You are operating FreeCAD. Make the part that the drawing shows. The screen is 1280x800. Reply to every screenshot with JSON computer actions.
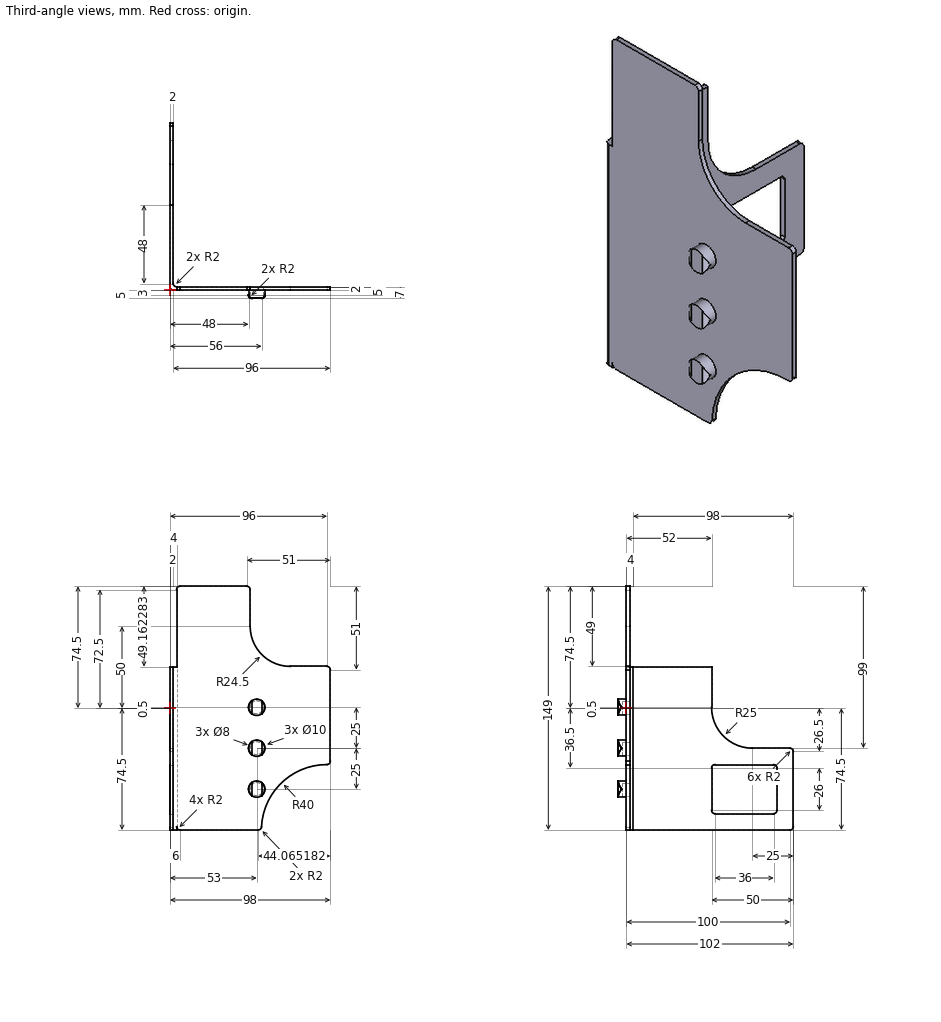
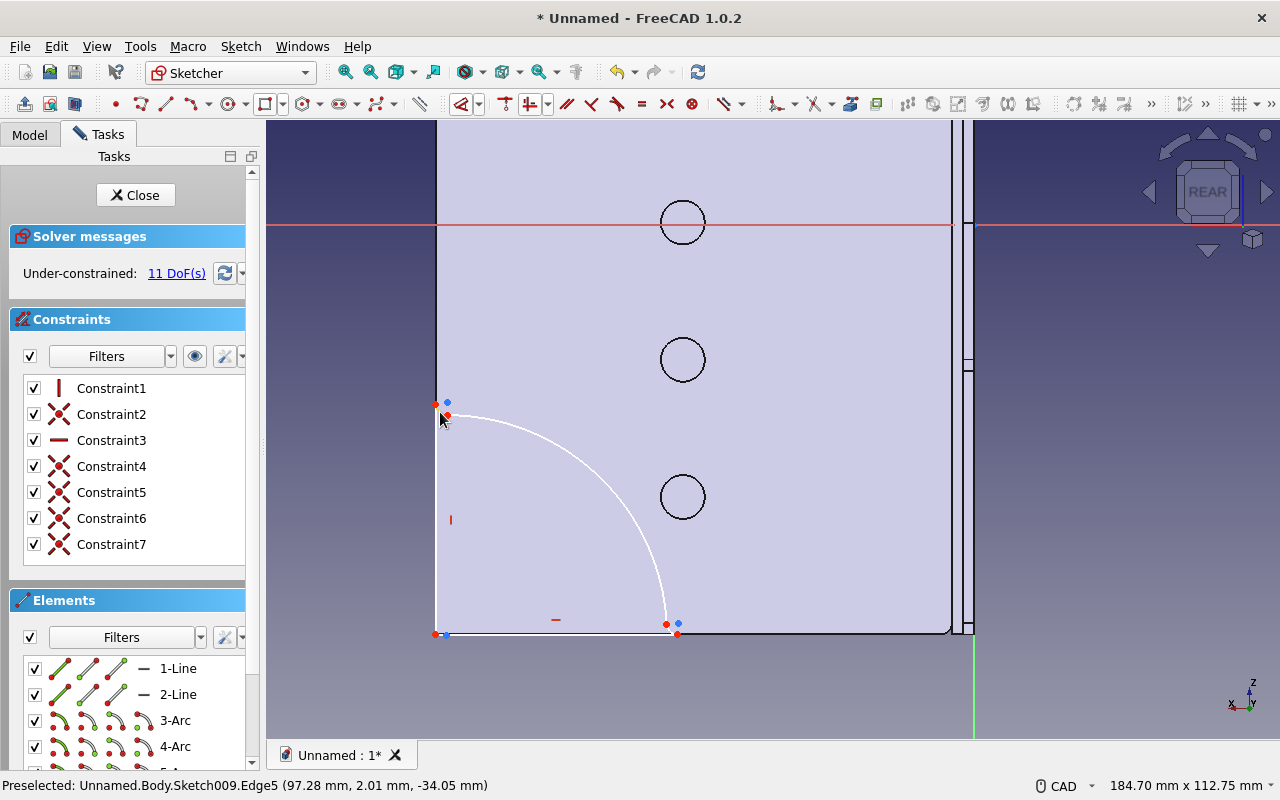
{"action": "left_click", "coordinate": [436, 451]}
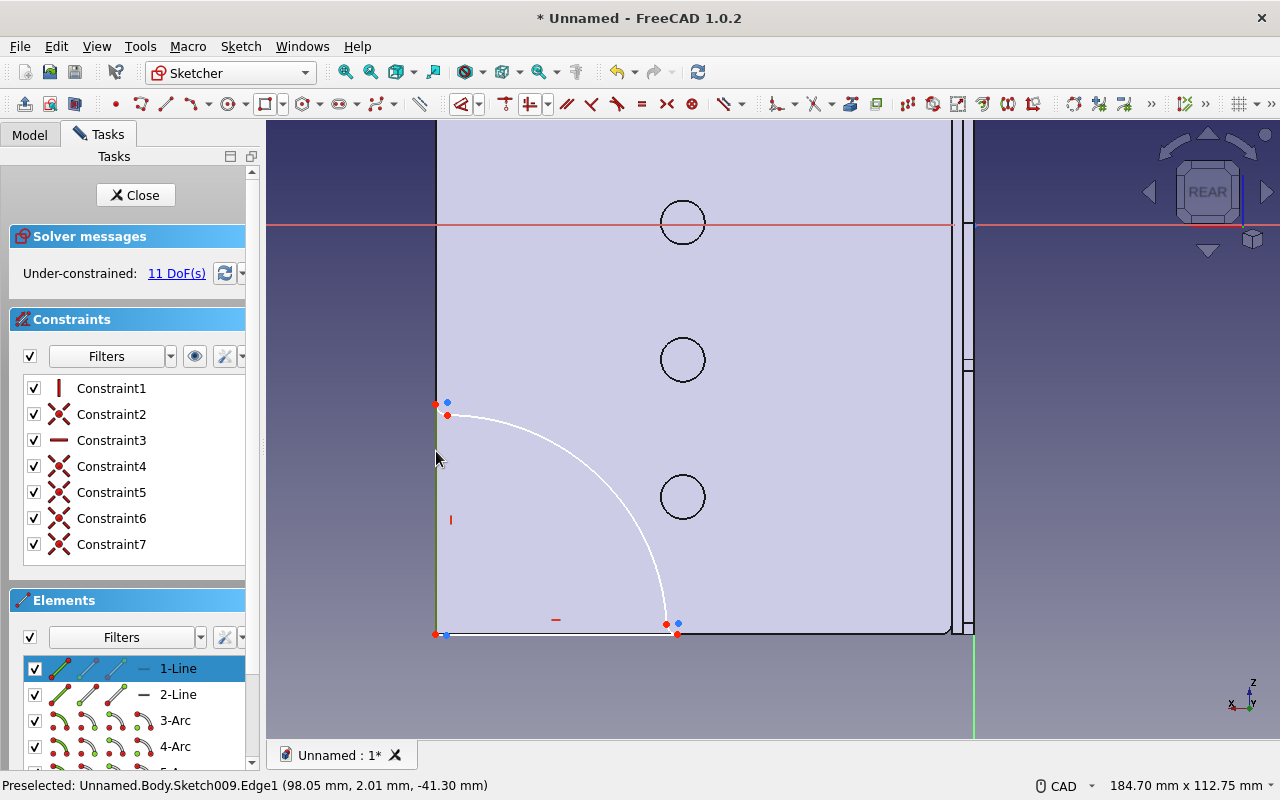
{"action": "scroll", "coordinate": [442, 414], "scroll_direction": "up", "scroll_amount": 6}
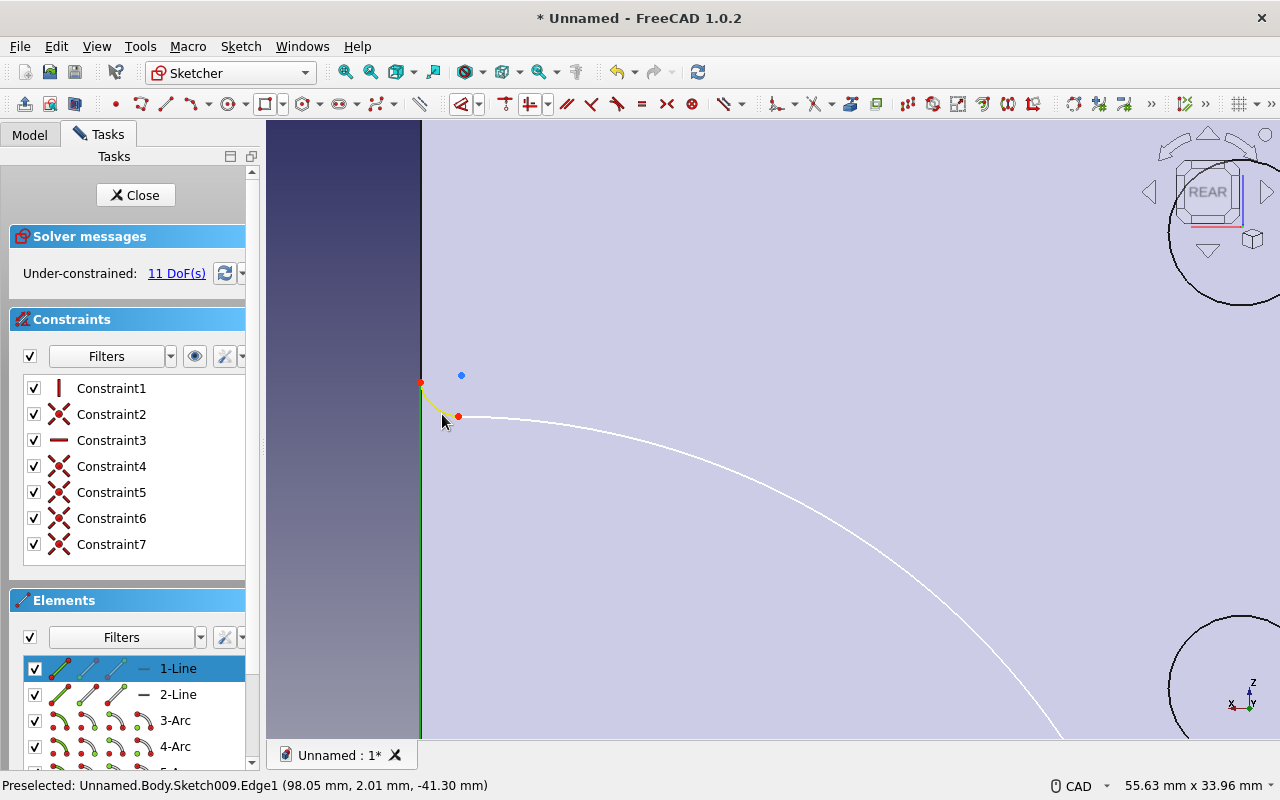
{"action": "left_click", "coordinate": [443, 412]}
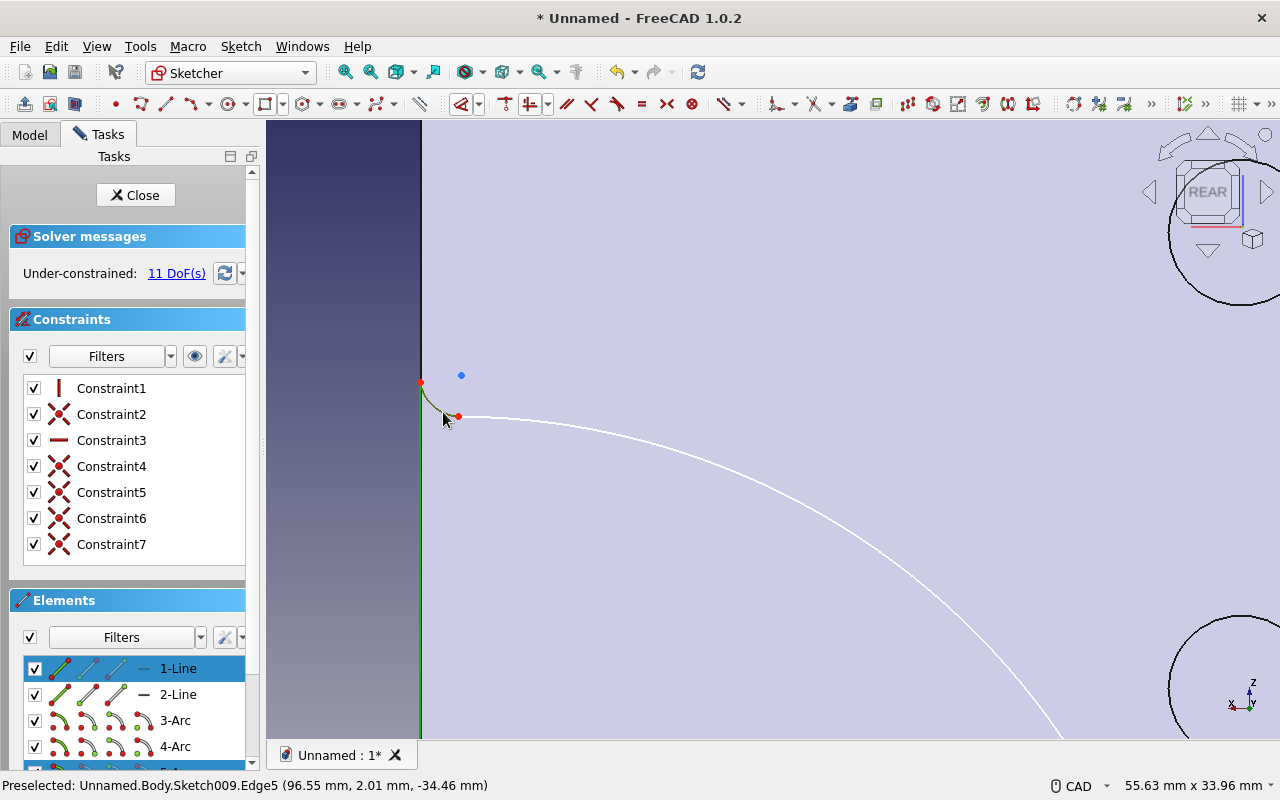
{"action": "key", "text": "t"}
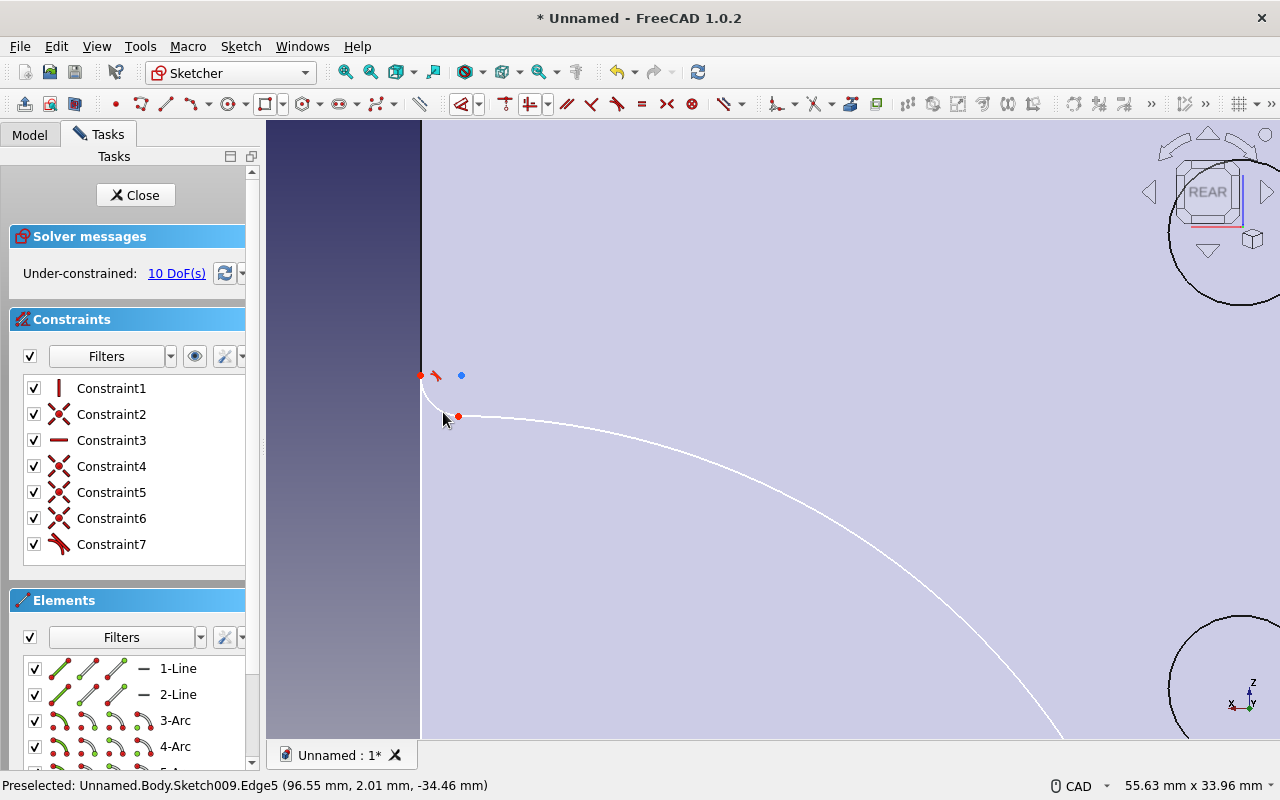
{"action": "scroll", "coordinate": [442, 414], "scroll_direction": "down", "scroll_amount": 6}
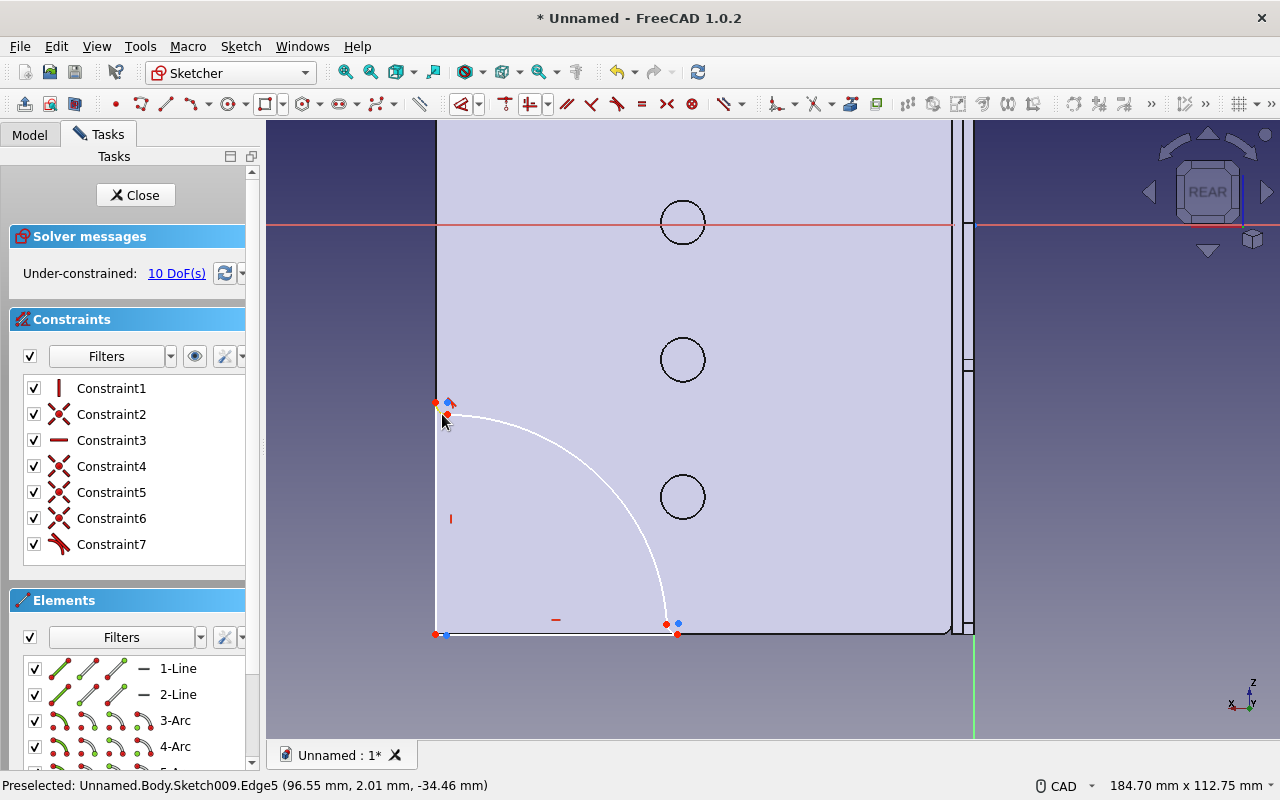
{"action": "left_click", "coordinate": [508, 635]}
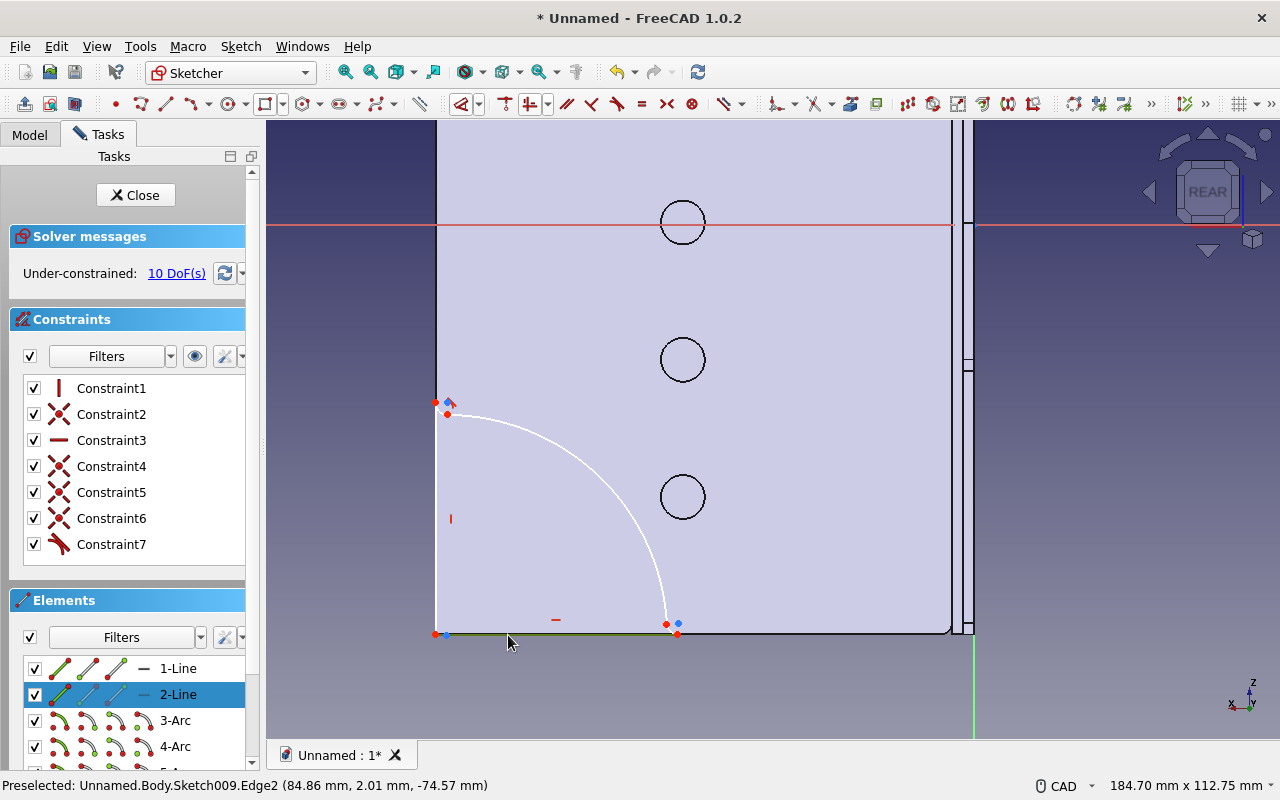
{"action": "scroll", "coordinate": [668, 629], "scroll_direction": "up", "scroll_amount": 6}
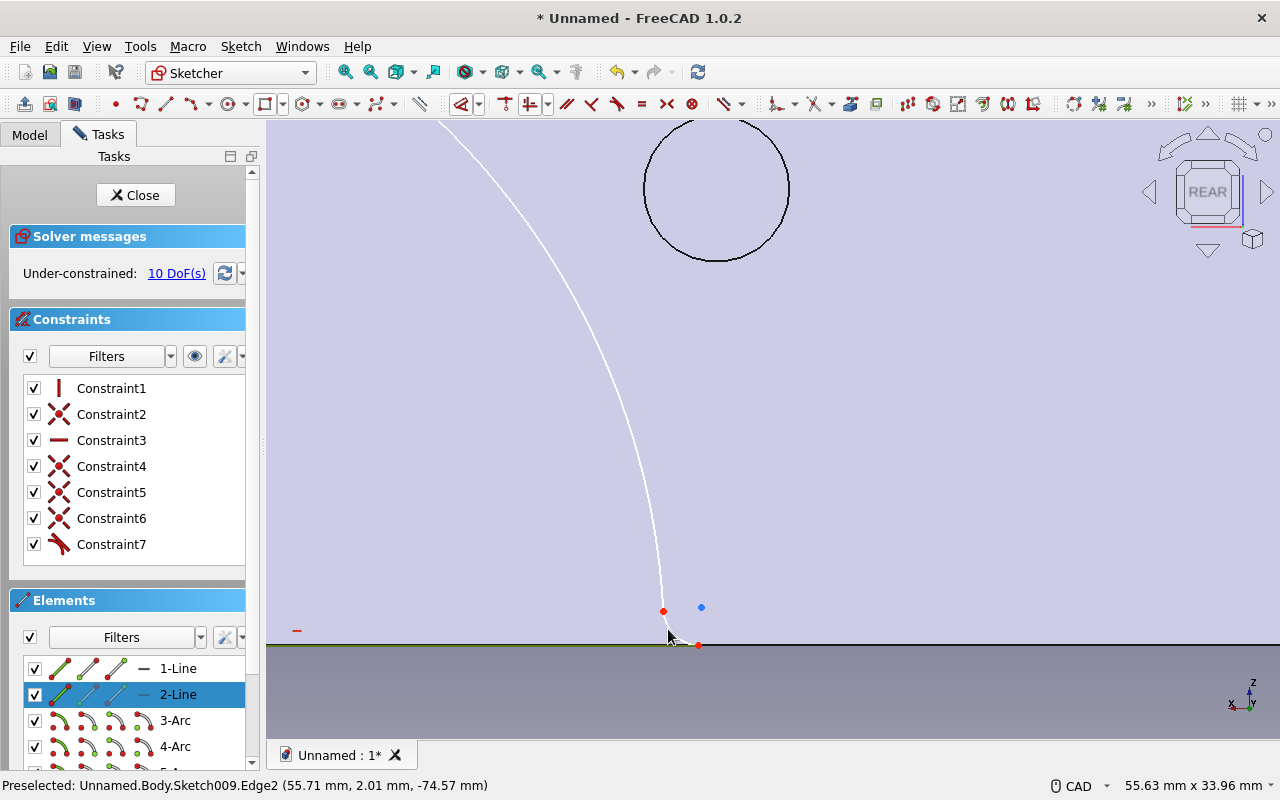
{"action": "left_click", "coordinate": [668, 626]}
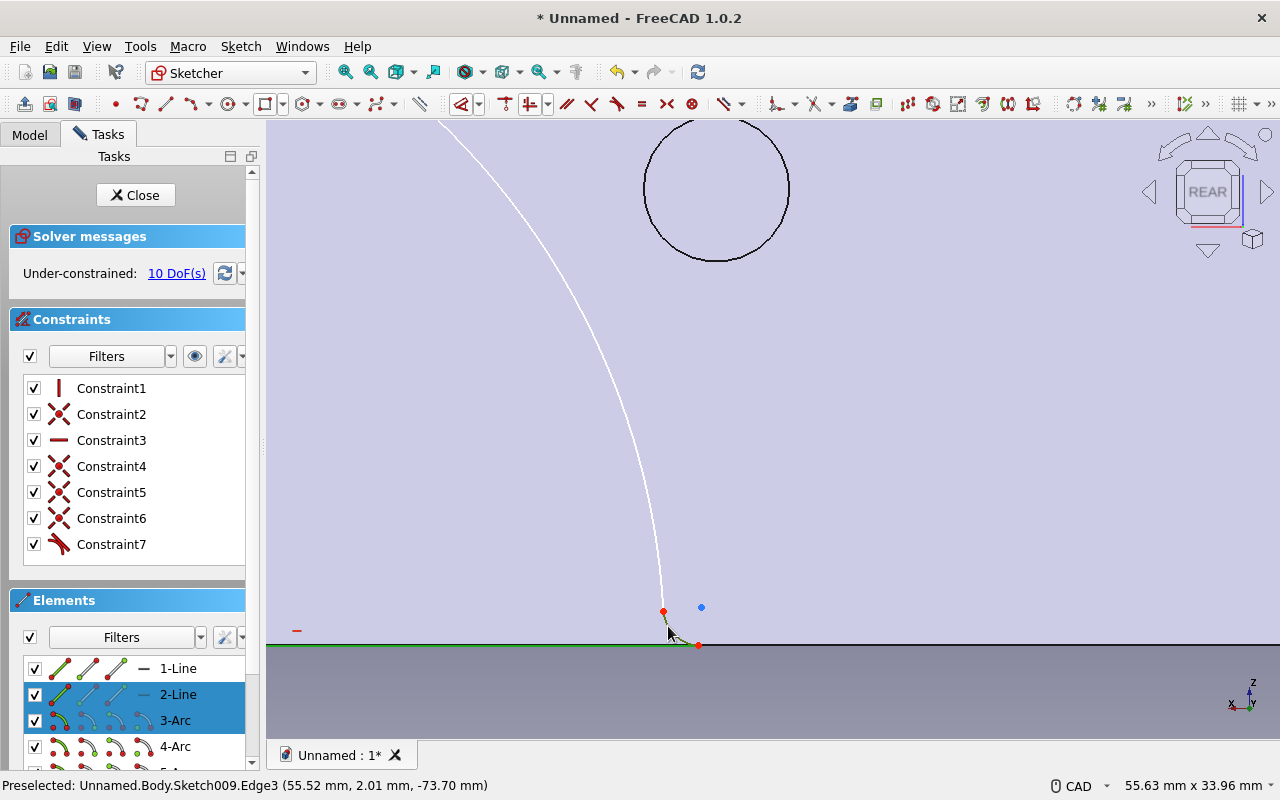
{"action": "key", "text": "t"}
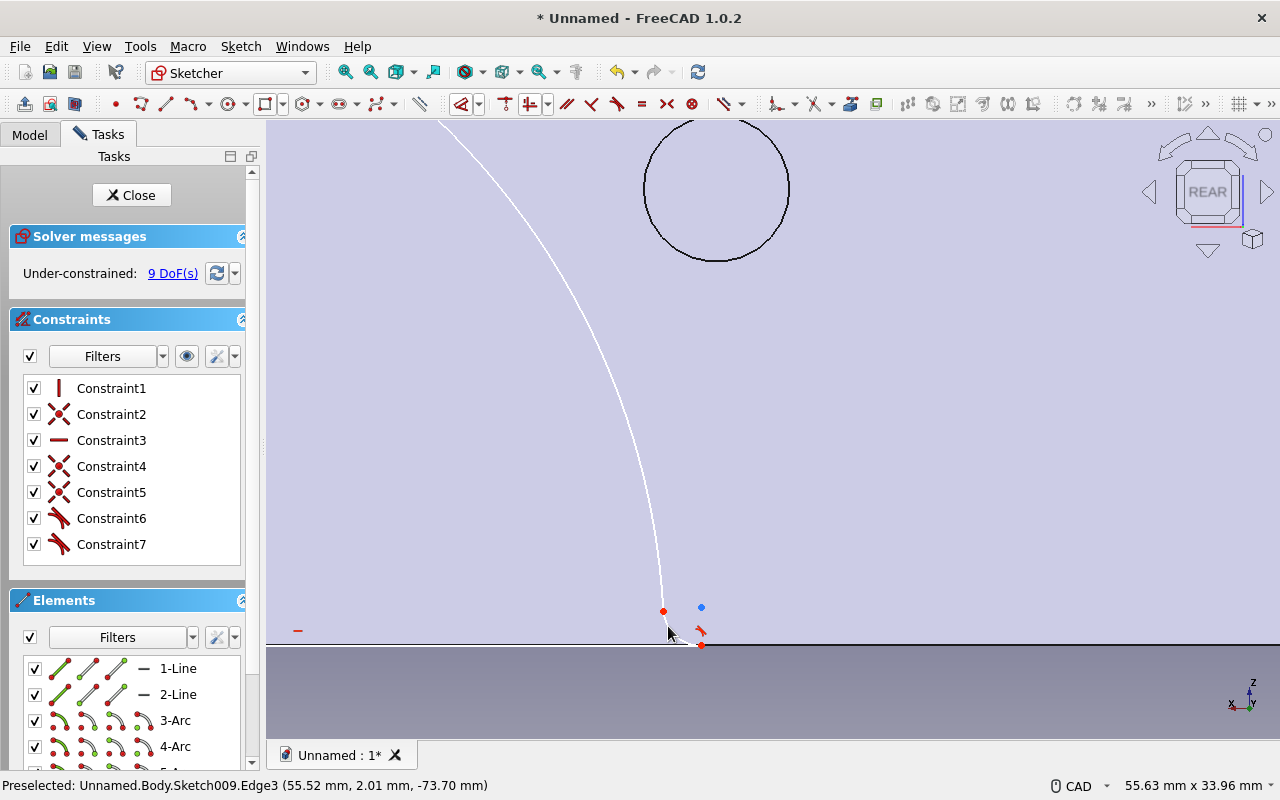
{"action": "left_click", "coordinate": [669, 627]}